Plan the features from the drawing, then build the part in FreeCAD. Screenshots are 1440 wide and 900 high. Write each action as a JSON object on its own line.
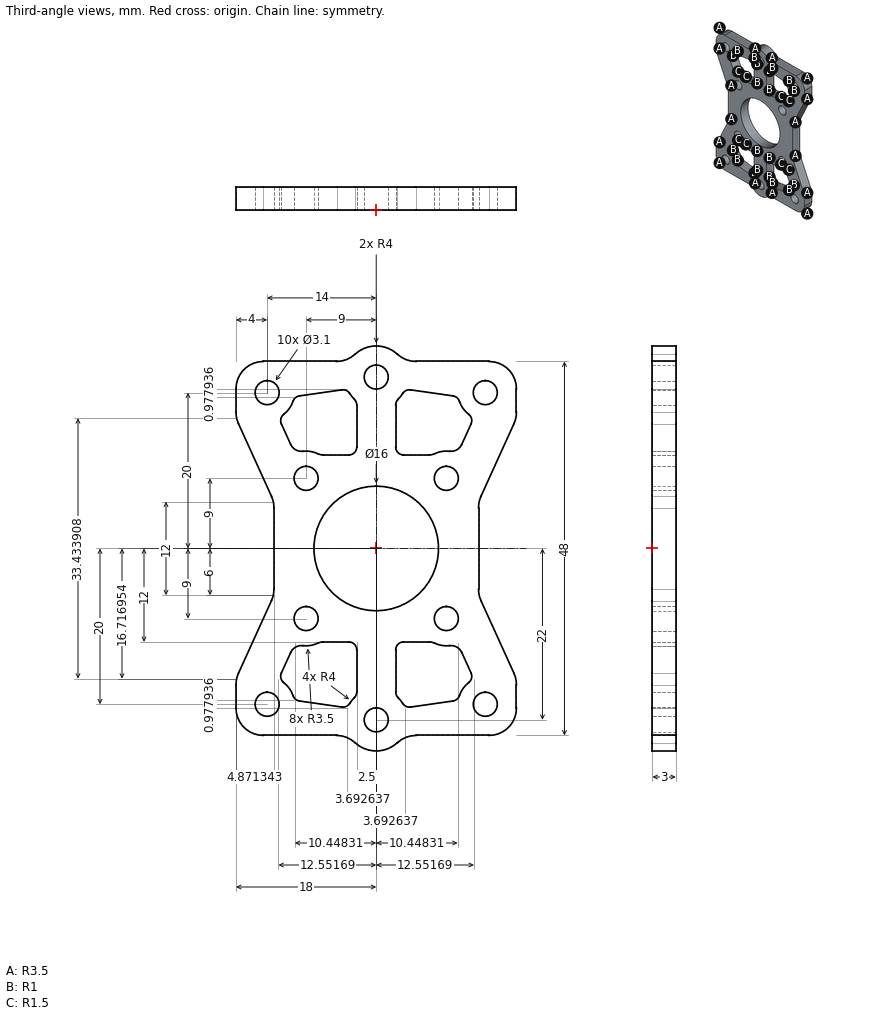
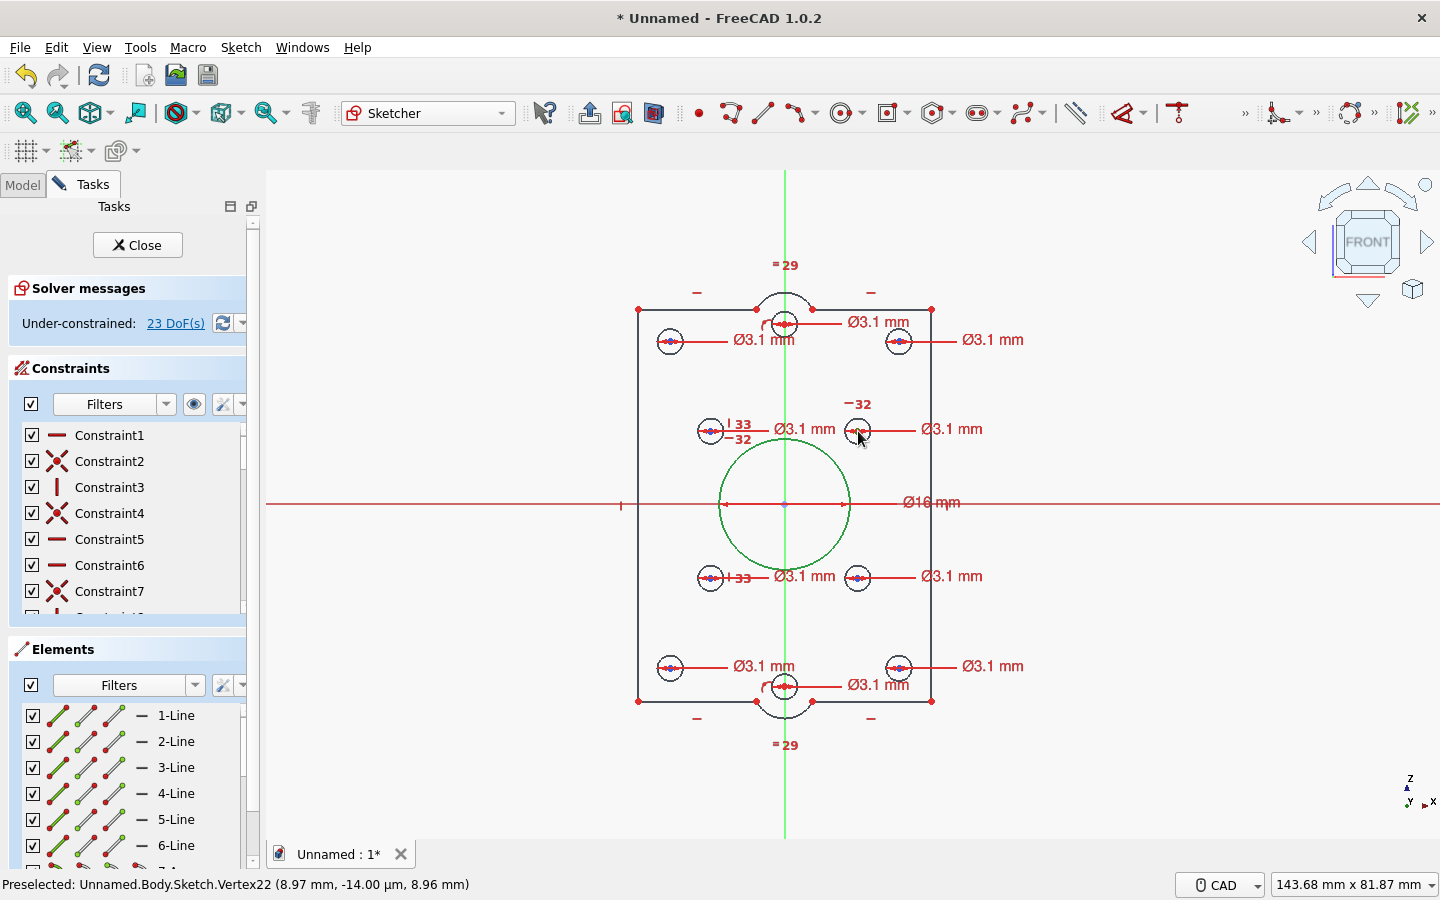
{"action": "left_click", "coordinate": [858, 578]}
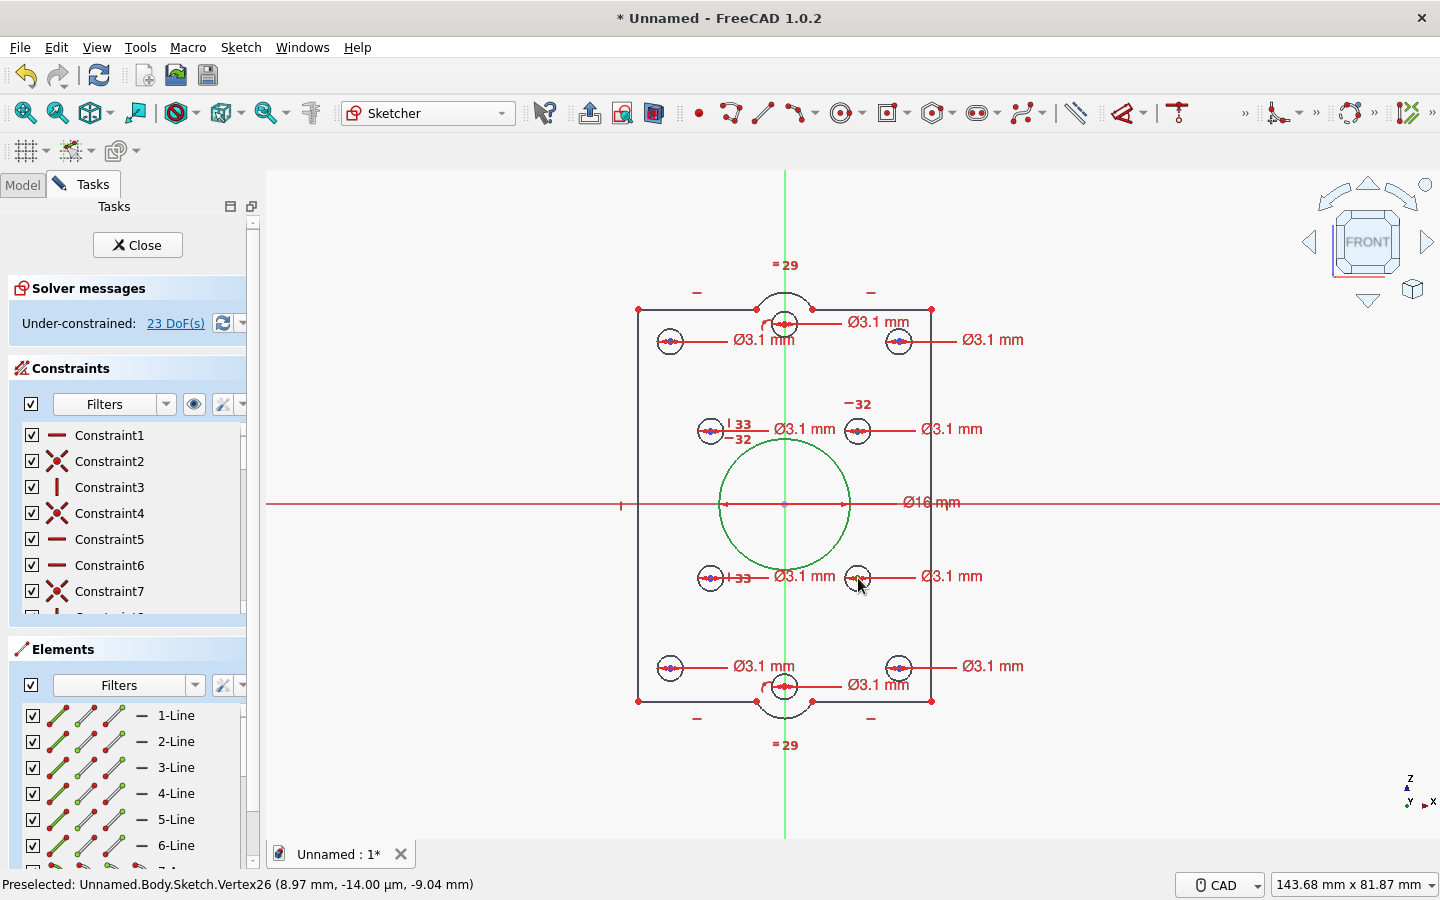
{"action": "key", "text": "v"}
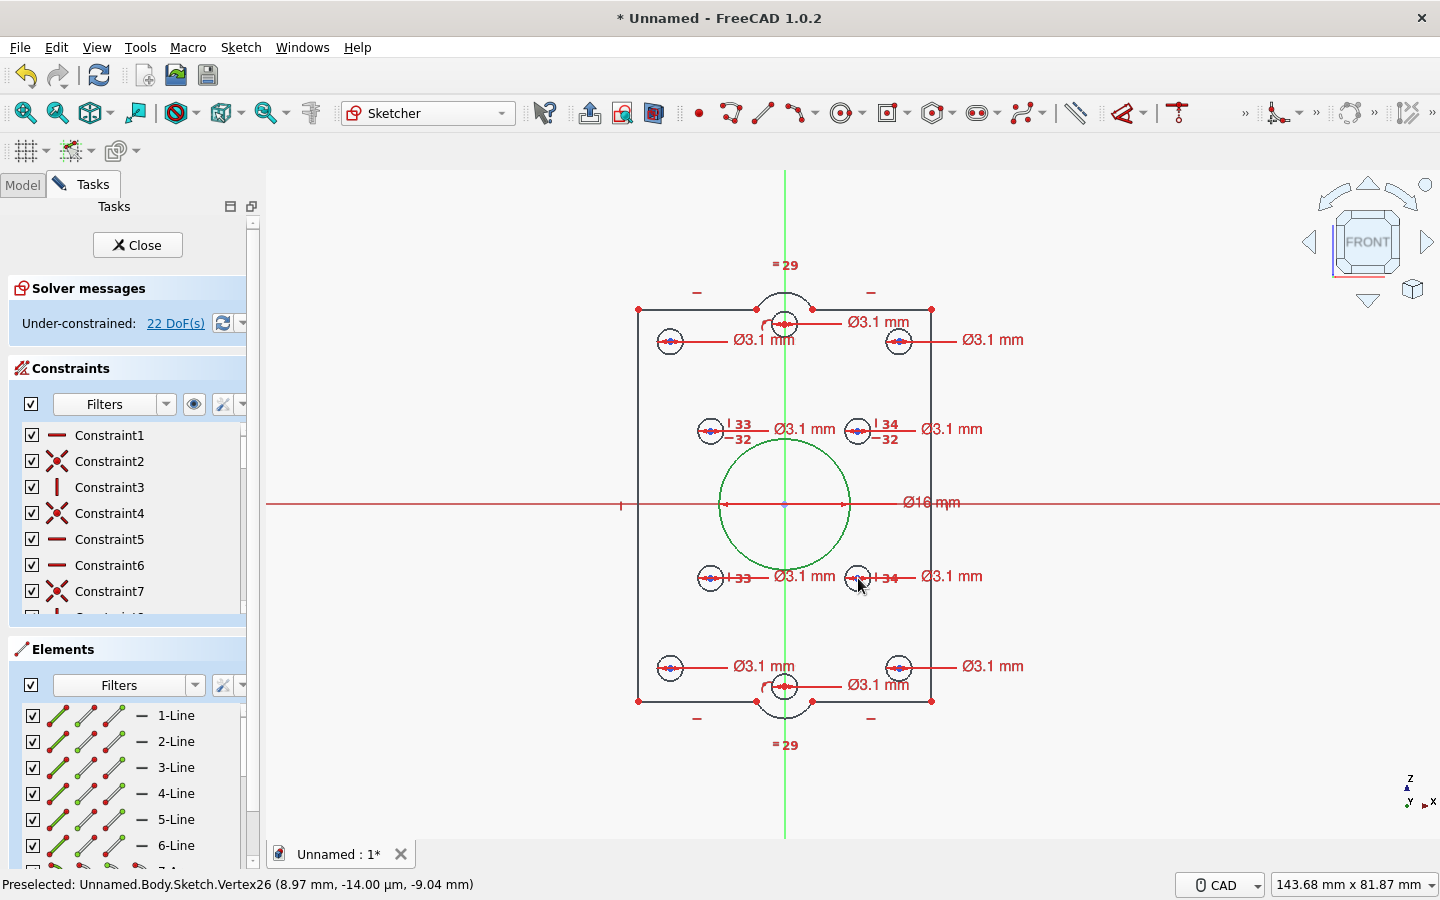
{"action": "left_click", "coordinate": [670, 342]}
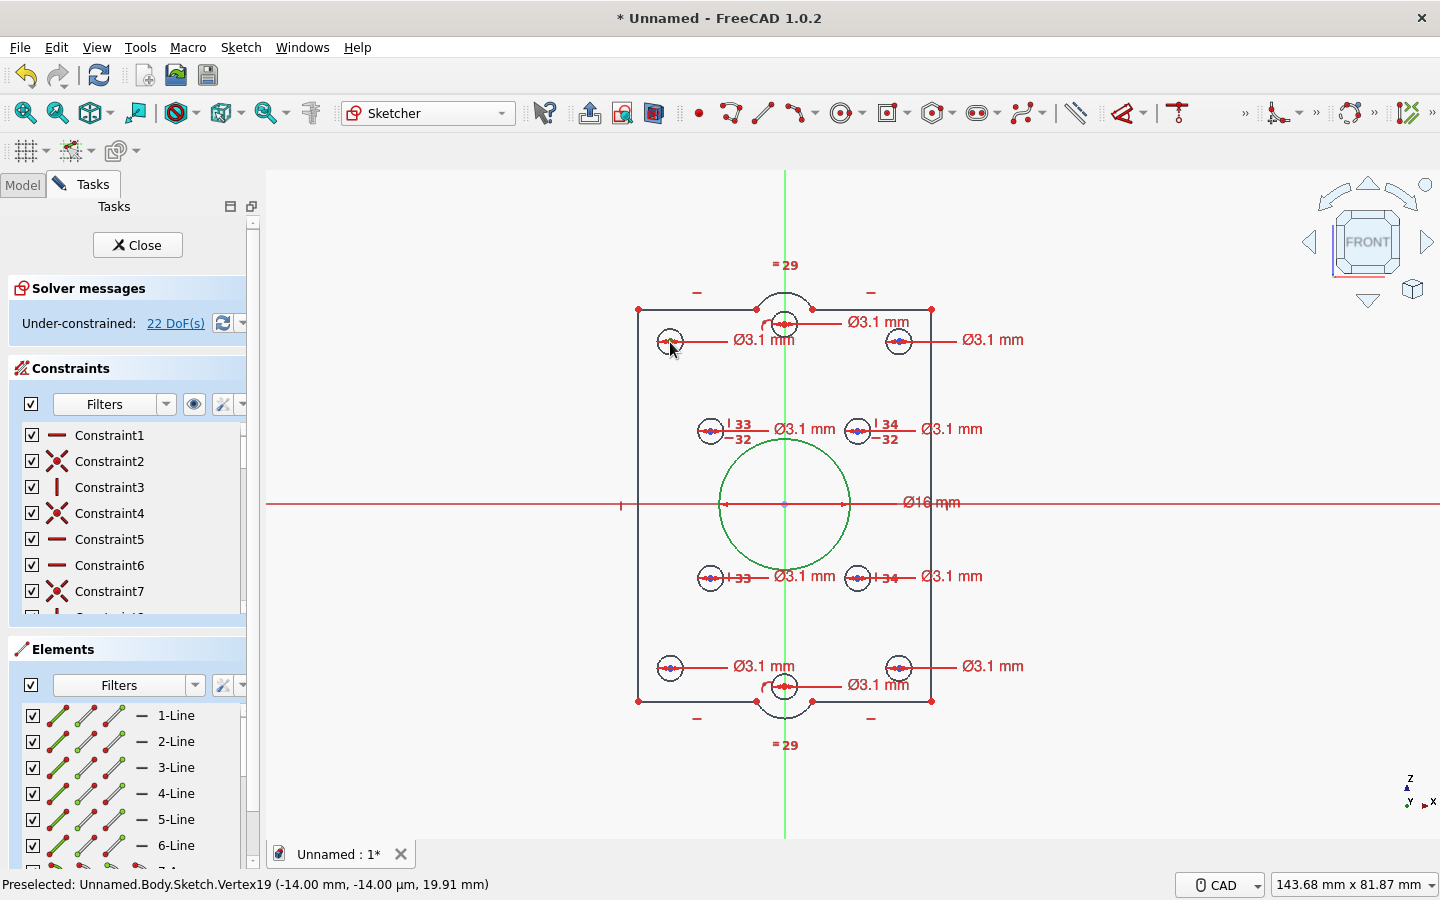
{"action": "left_click", "coordinate": [899, 342]}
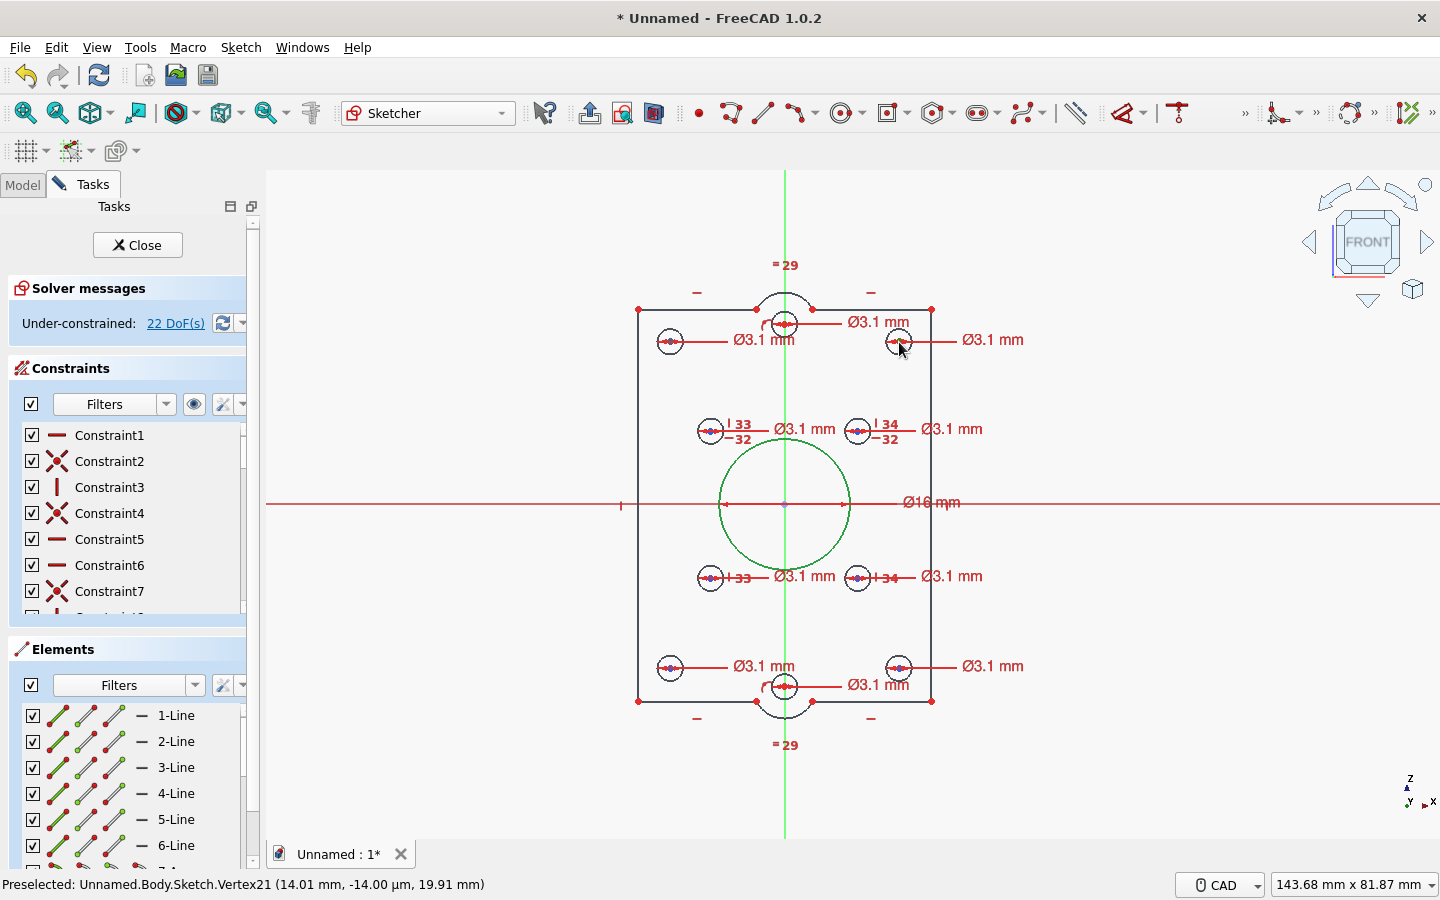
{"action": "left_click", "coordinate": [785, 767]}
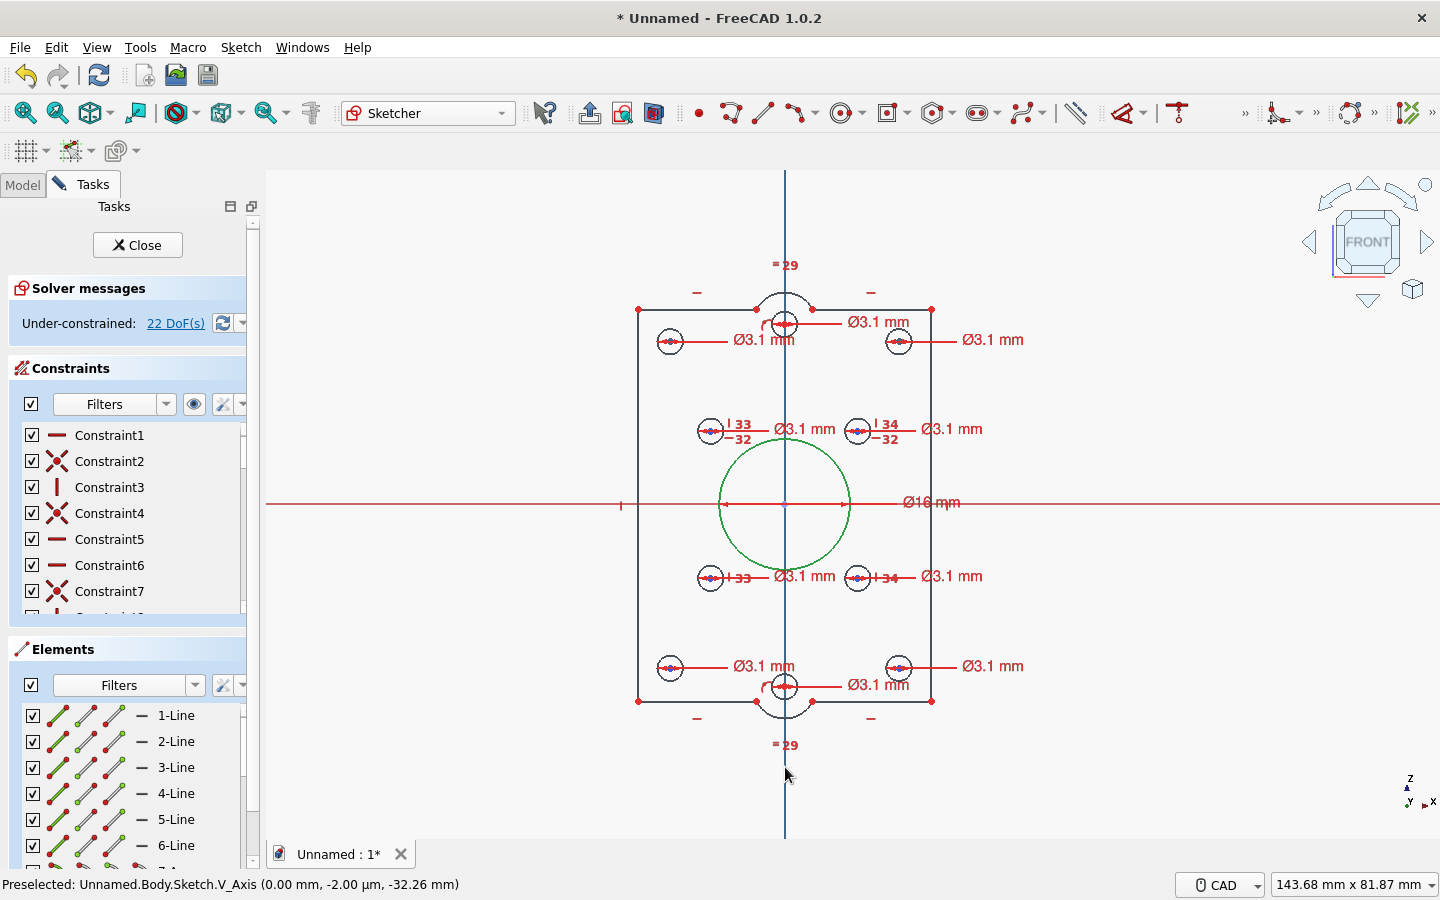
{"action": "key", "text": "s"}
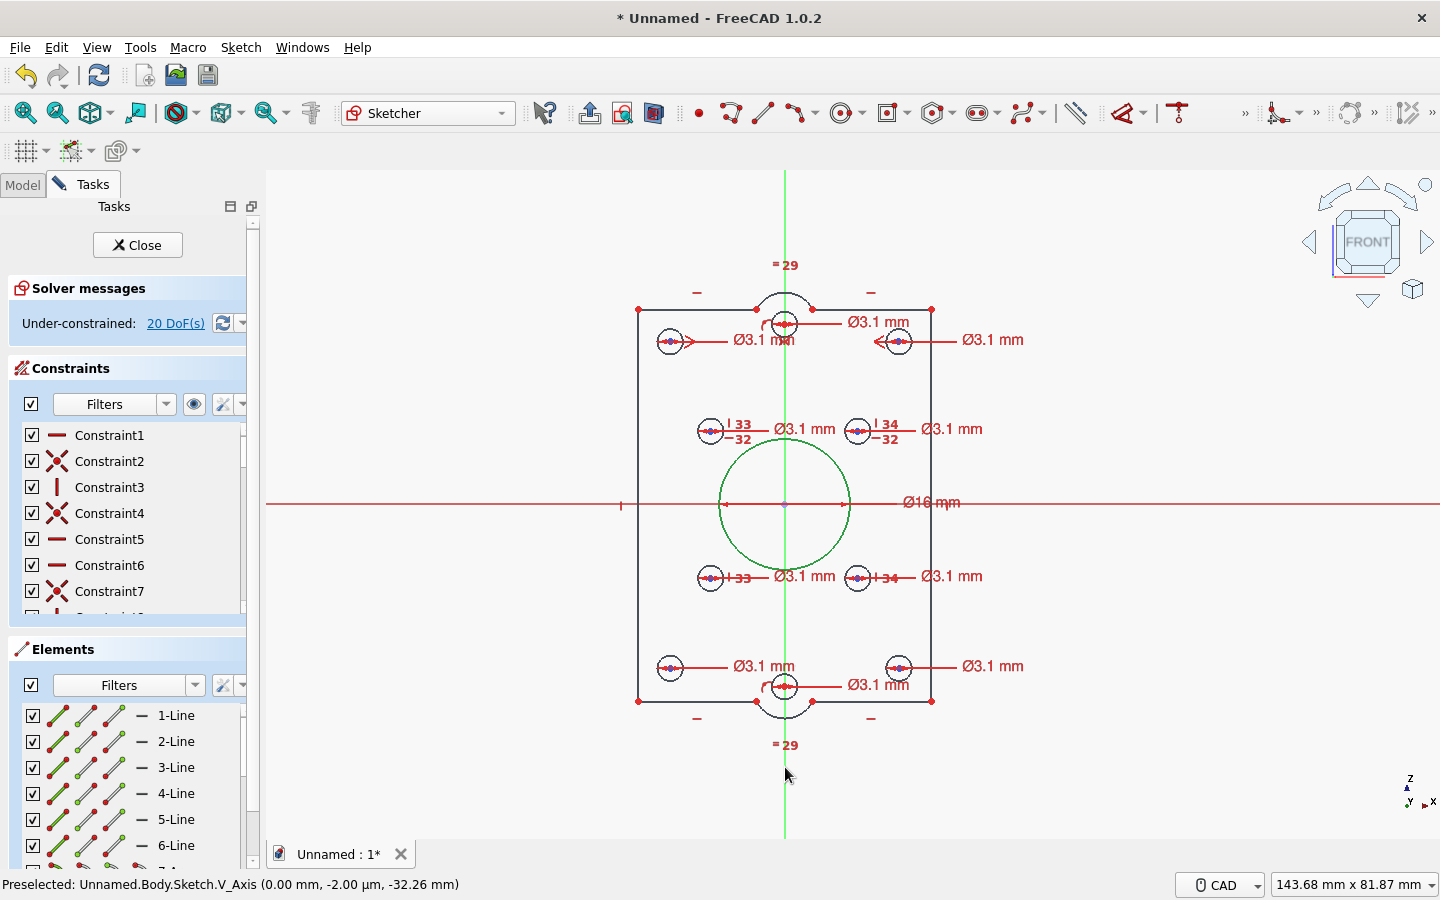
{"action": "left_click", "coordinate": [670, 342]}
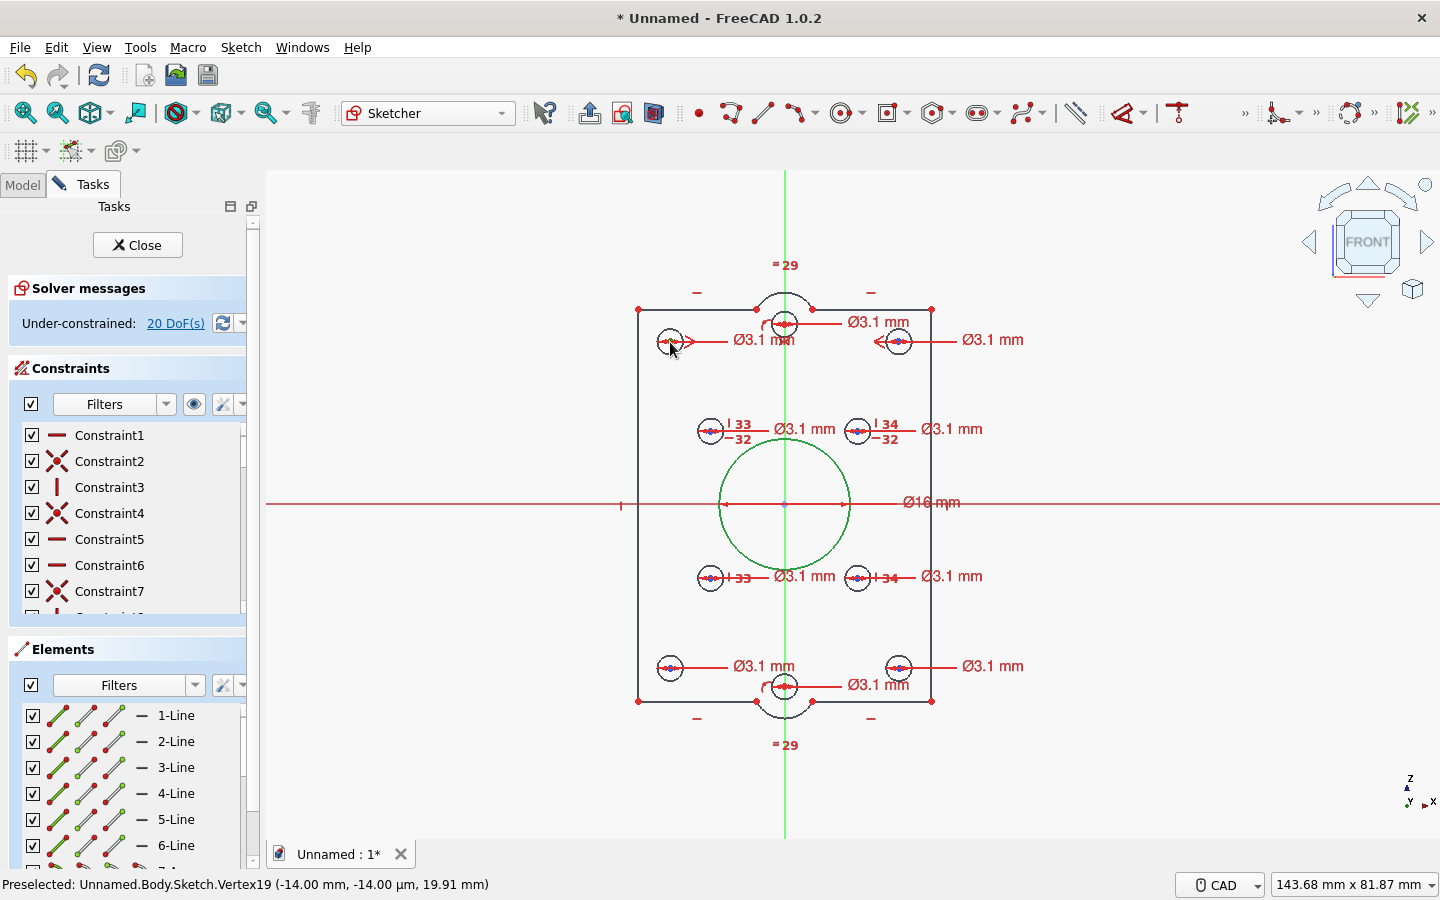
{"action": "left_click", "coordinate": [670, 668]}